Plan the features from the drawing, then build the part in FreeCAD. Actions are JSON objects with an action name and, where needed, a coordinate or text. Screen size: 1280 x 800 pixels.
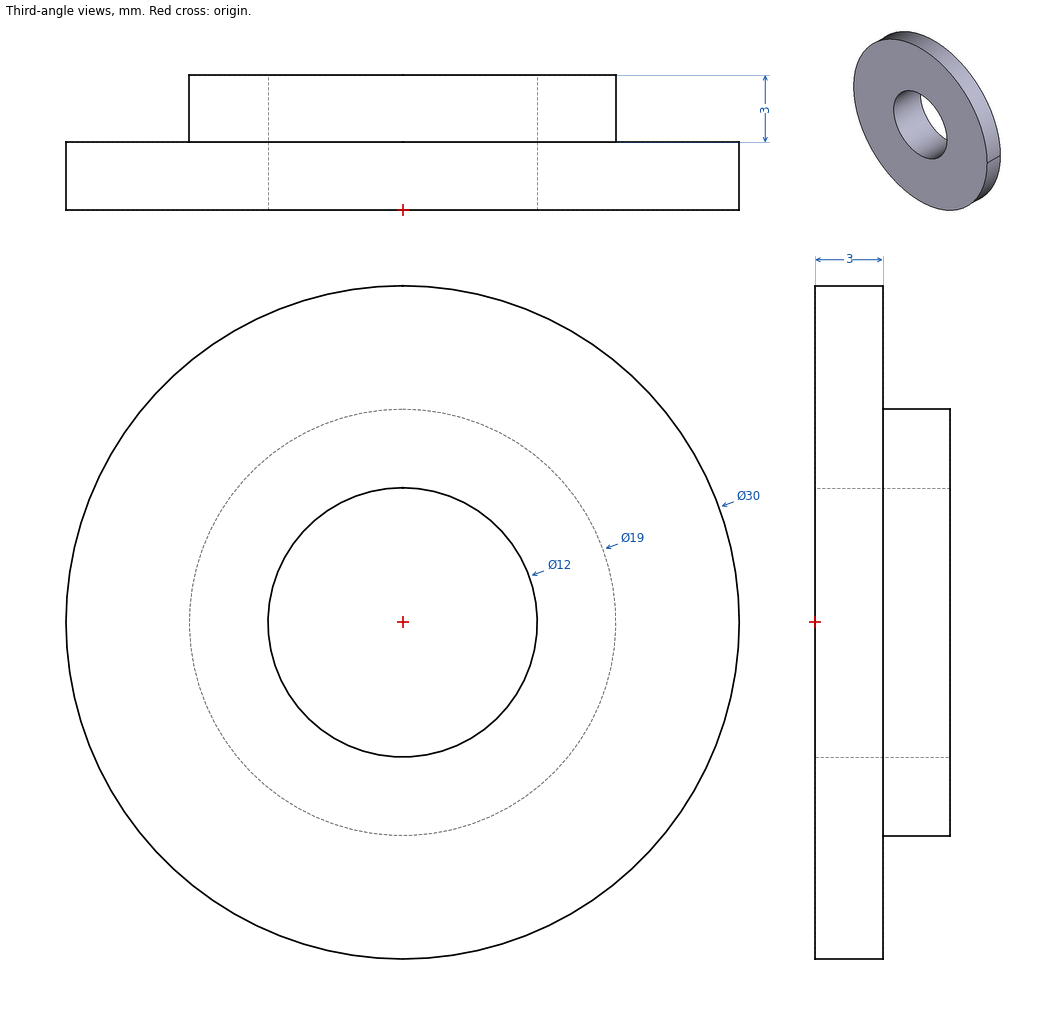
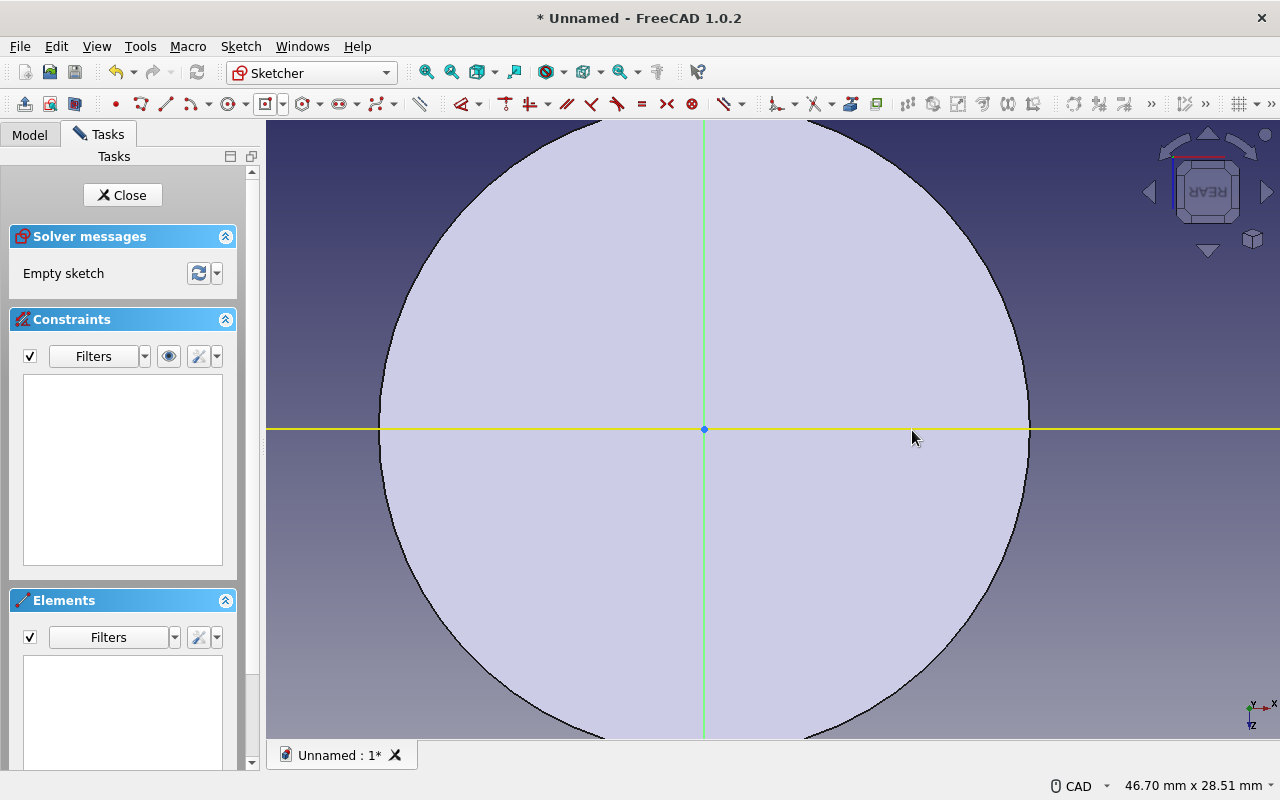
{"action": "left_click", "coordinate": [228, 104]}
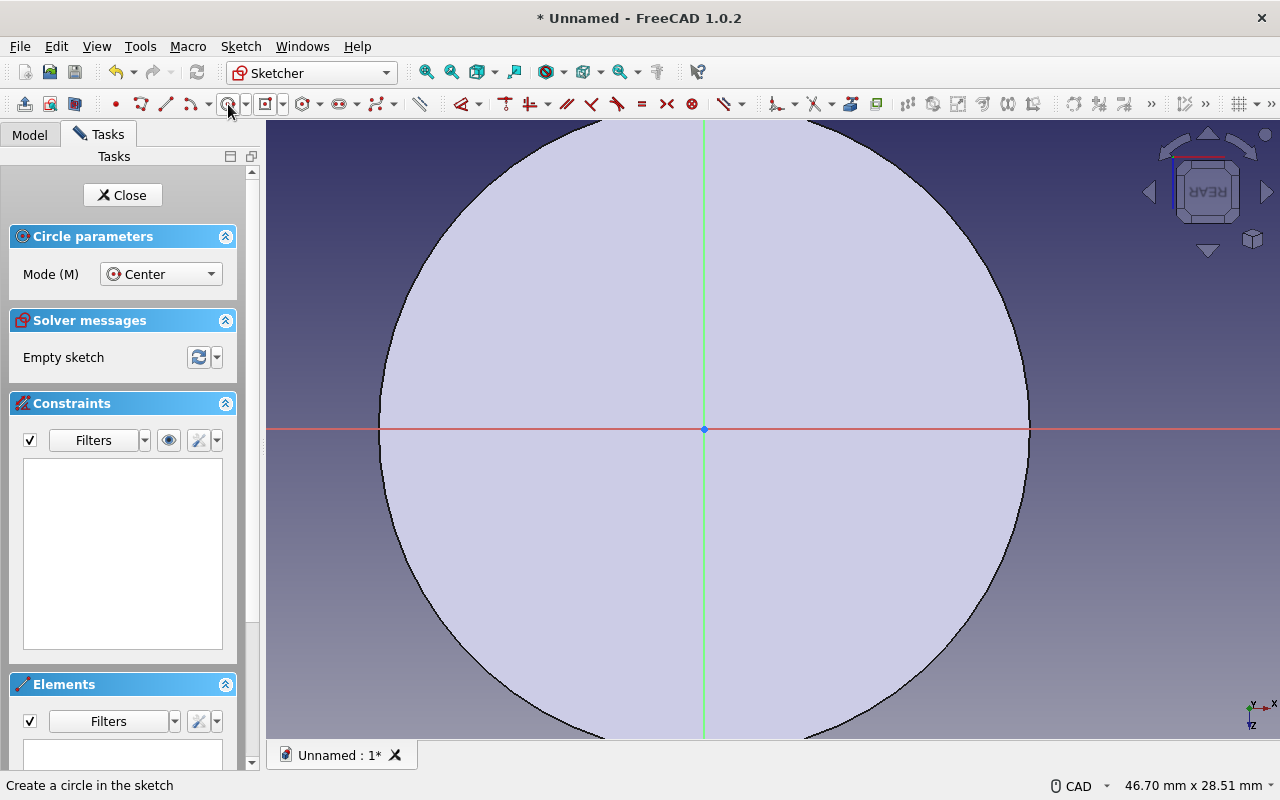
{"action": "left_click", "coordinate": [704, 429]}
{"action": "left_click", "coordinate": [850, 283]}
{"action": "key", "text": "Escape"}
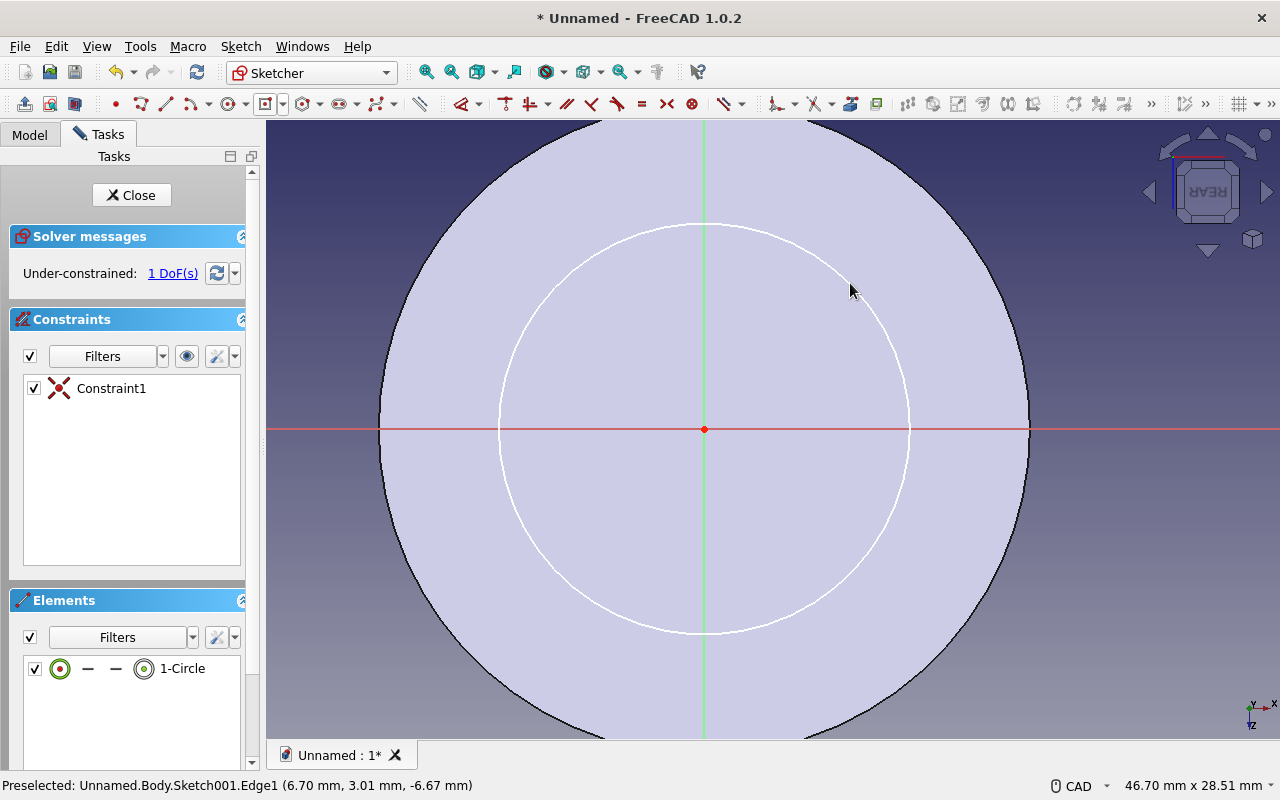
{"action": "left_click", "coordinate": [460, 104]}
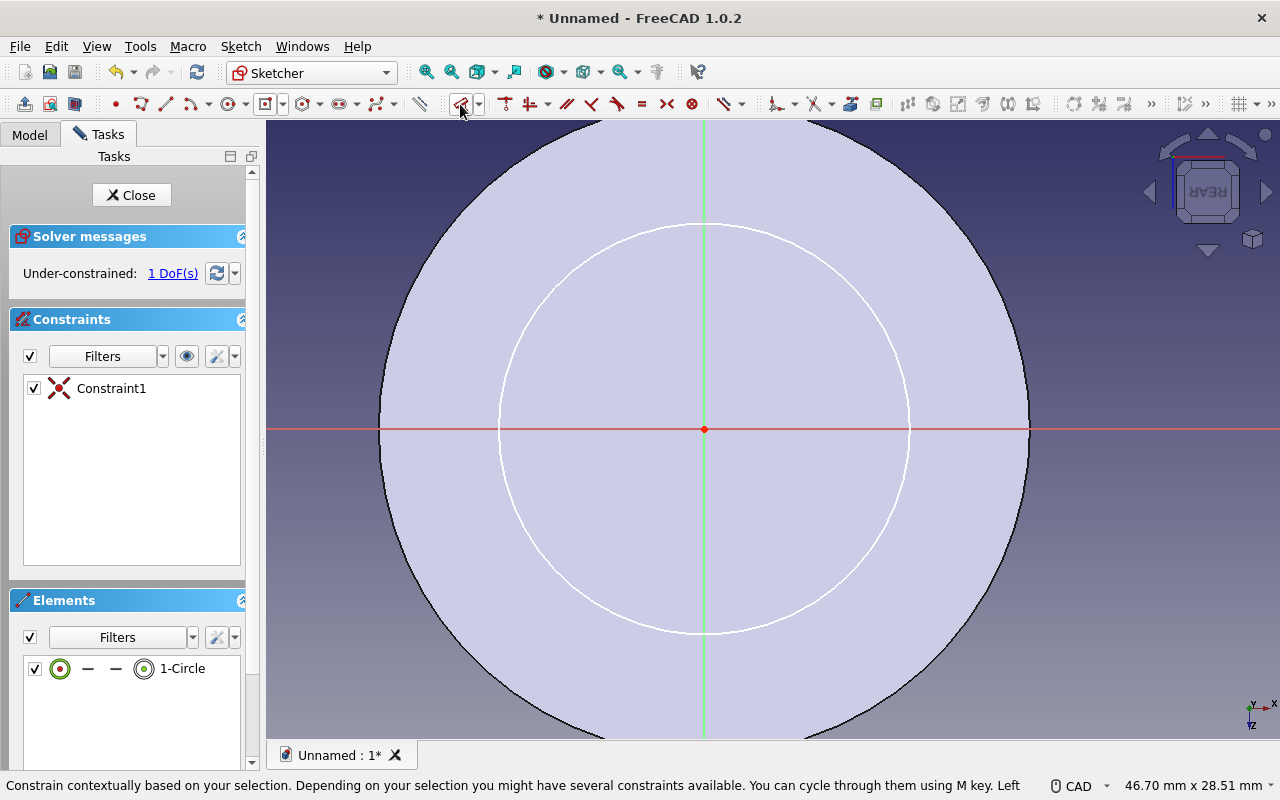
{"action": "left_click", "coordinate": [849, 283]}
{"action": "left_click", "coordinate": [872, 260]}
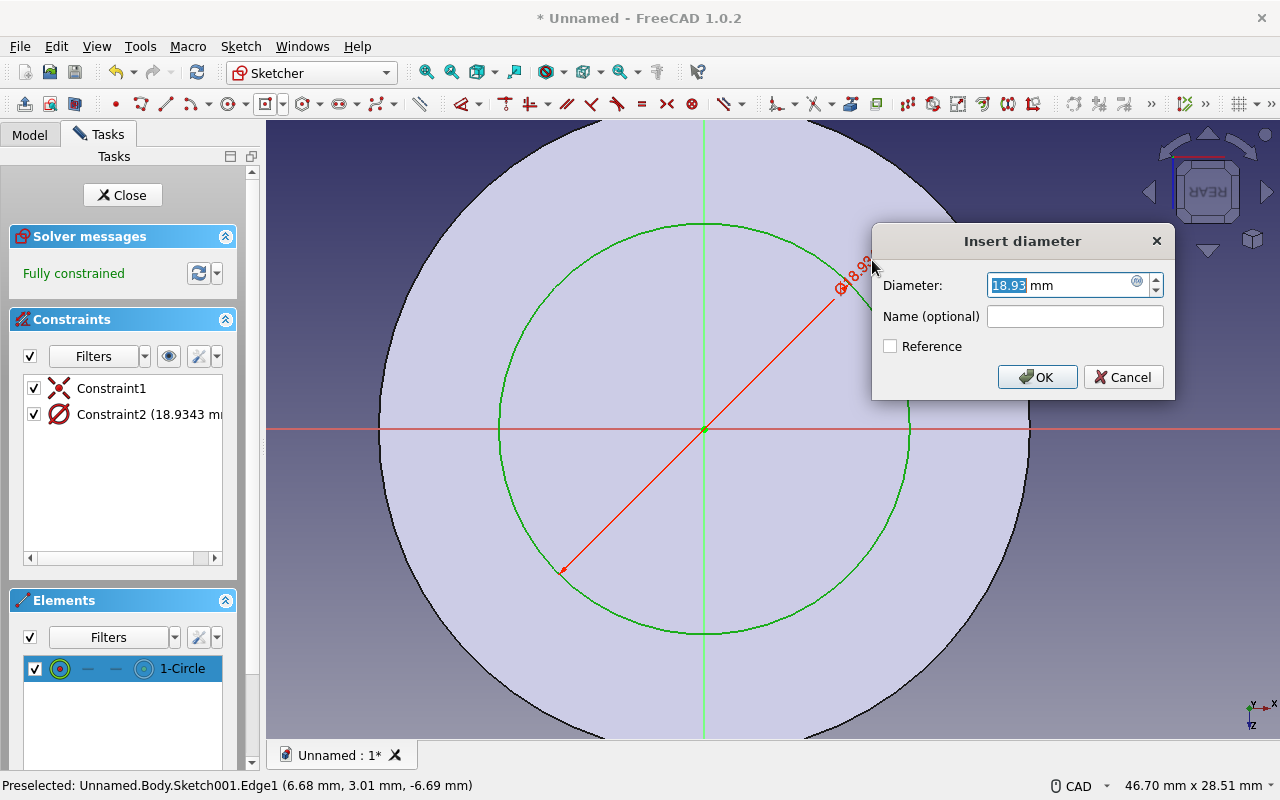
{"action": "type", "text": "19"}
{"action": "key", "text": "Return"}
{"action": "key", "text": "Escape"}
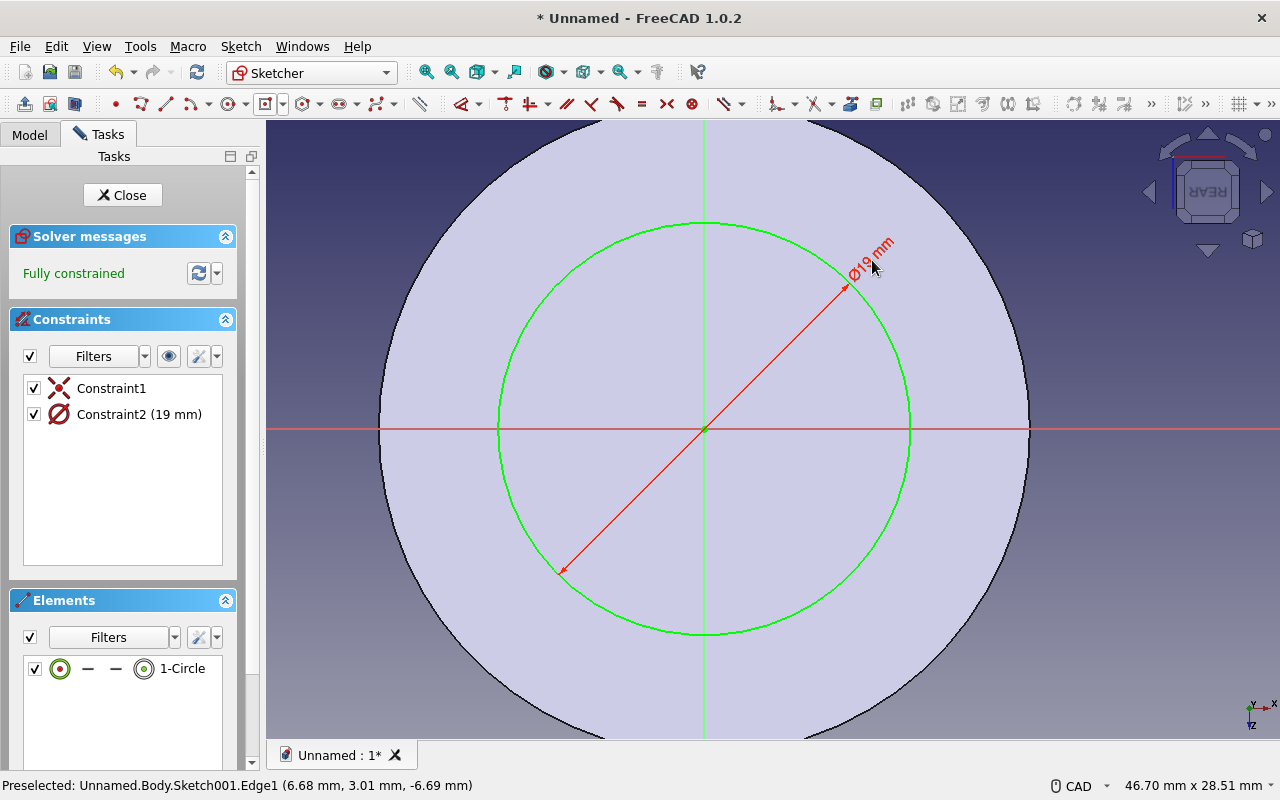
{"action": "left_click", "coordinate": [123, 195]}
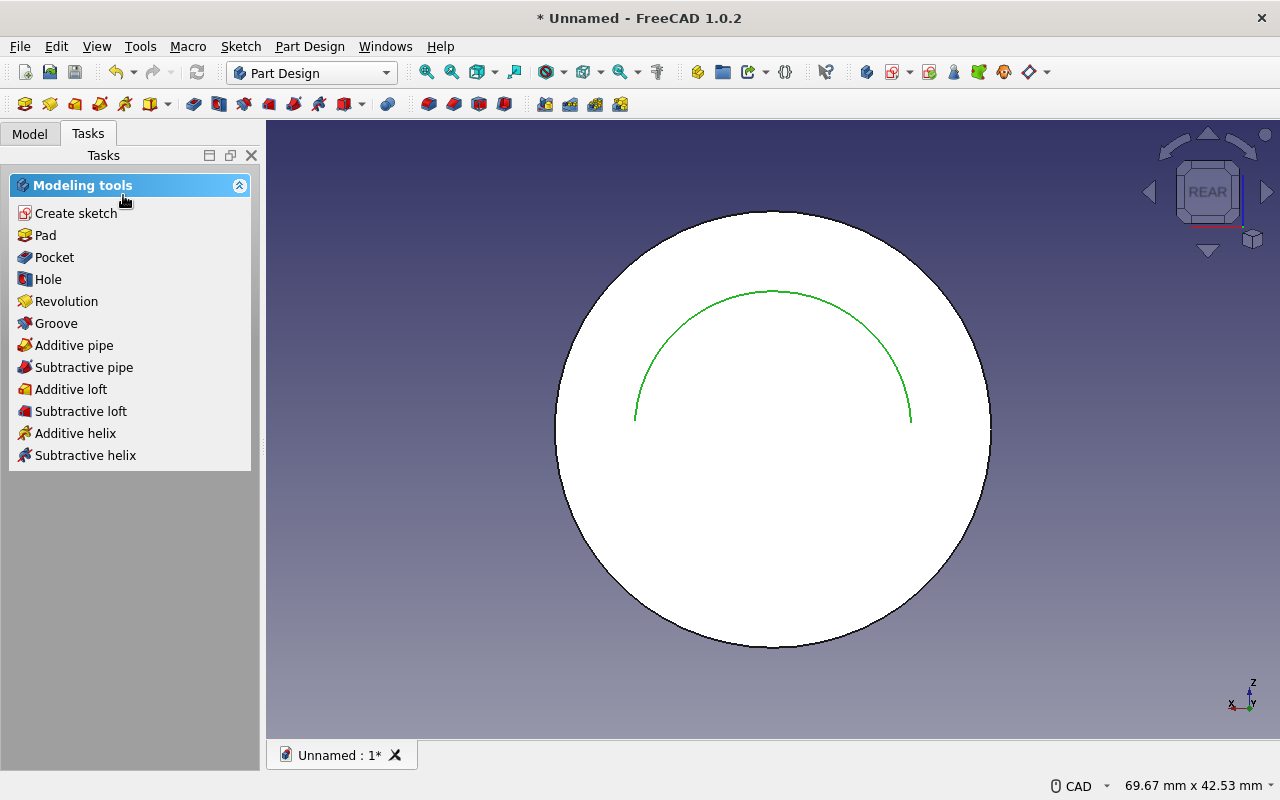
{"action": "left_click", "coordinate": [25, 104]}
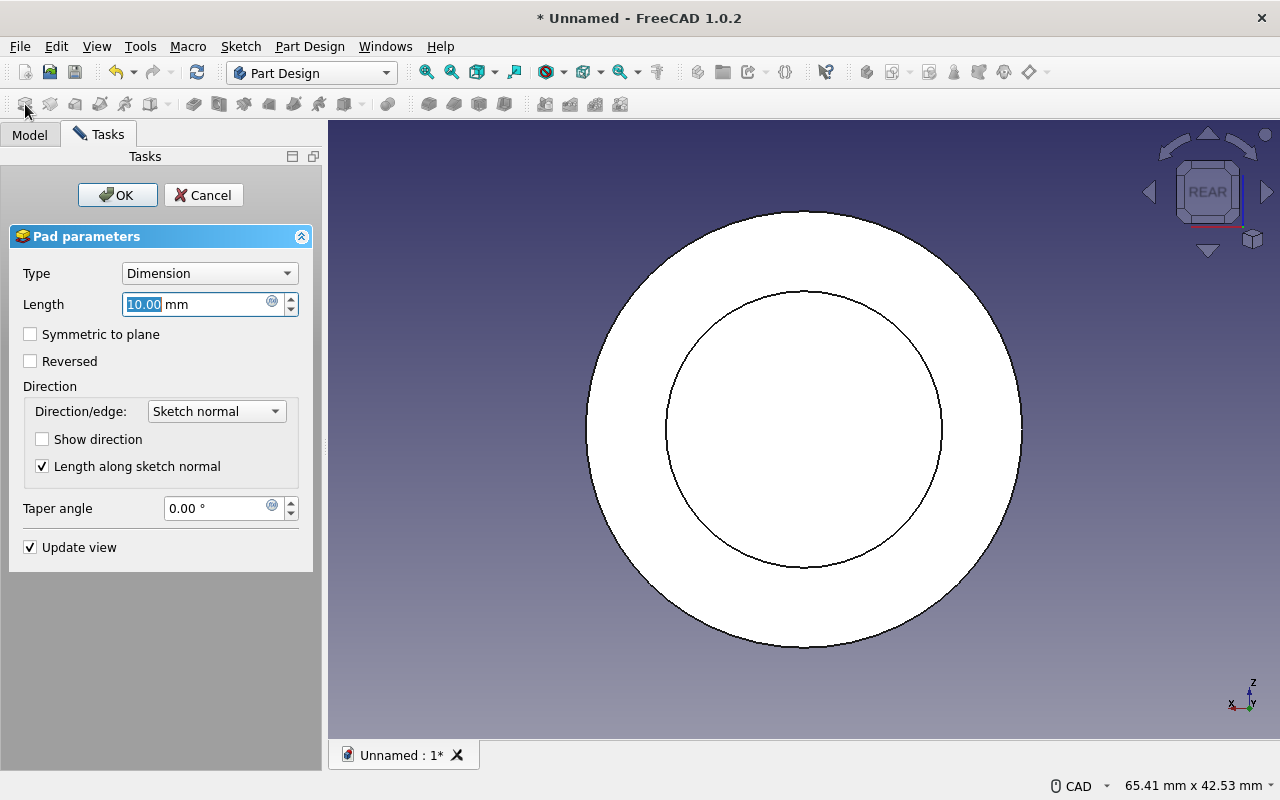
{"action": "type", "text": "3"}
{"action": "key", "text": "Tab"}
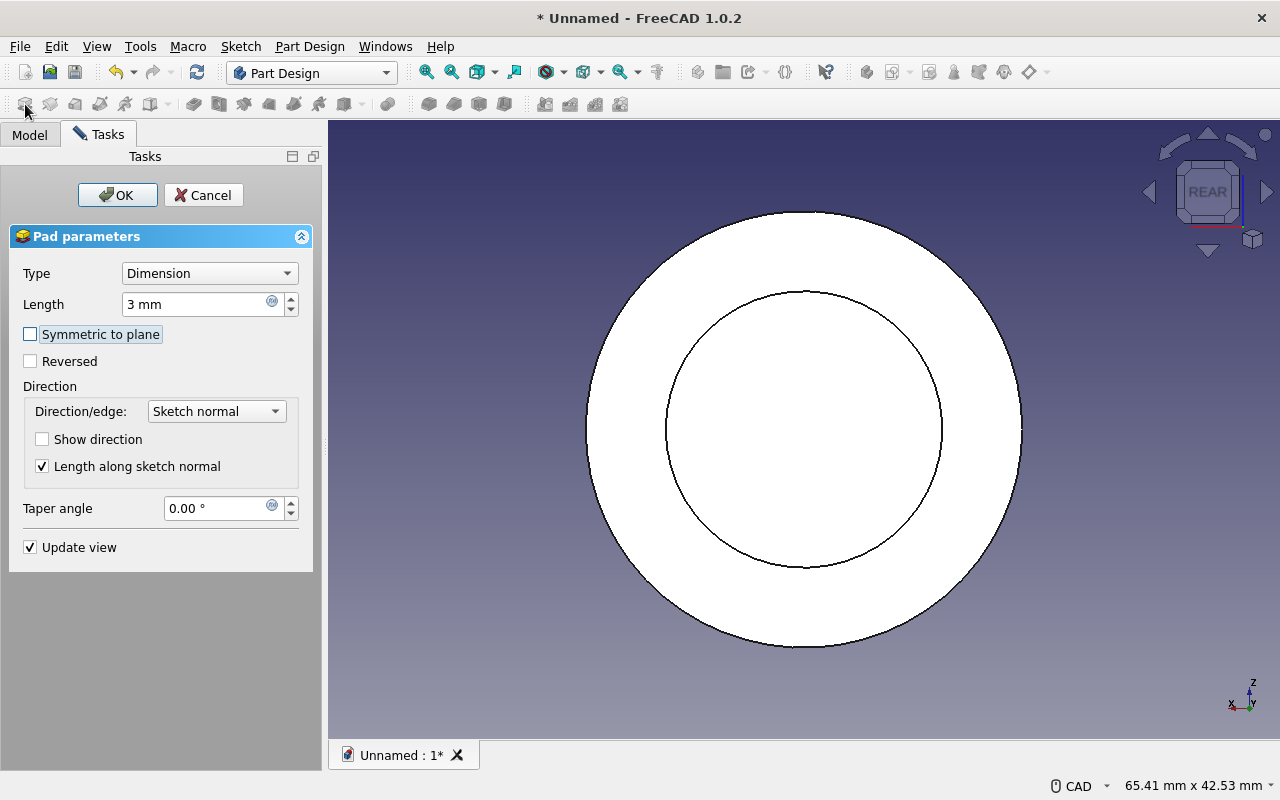
{"action": "left_click", "coordinate": [118, 195]}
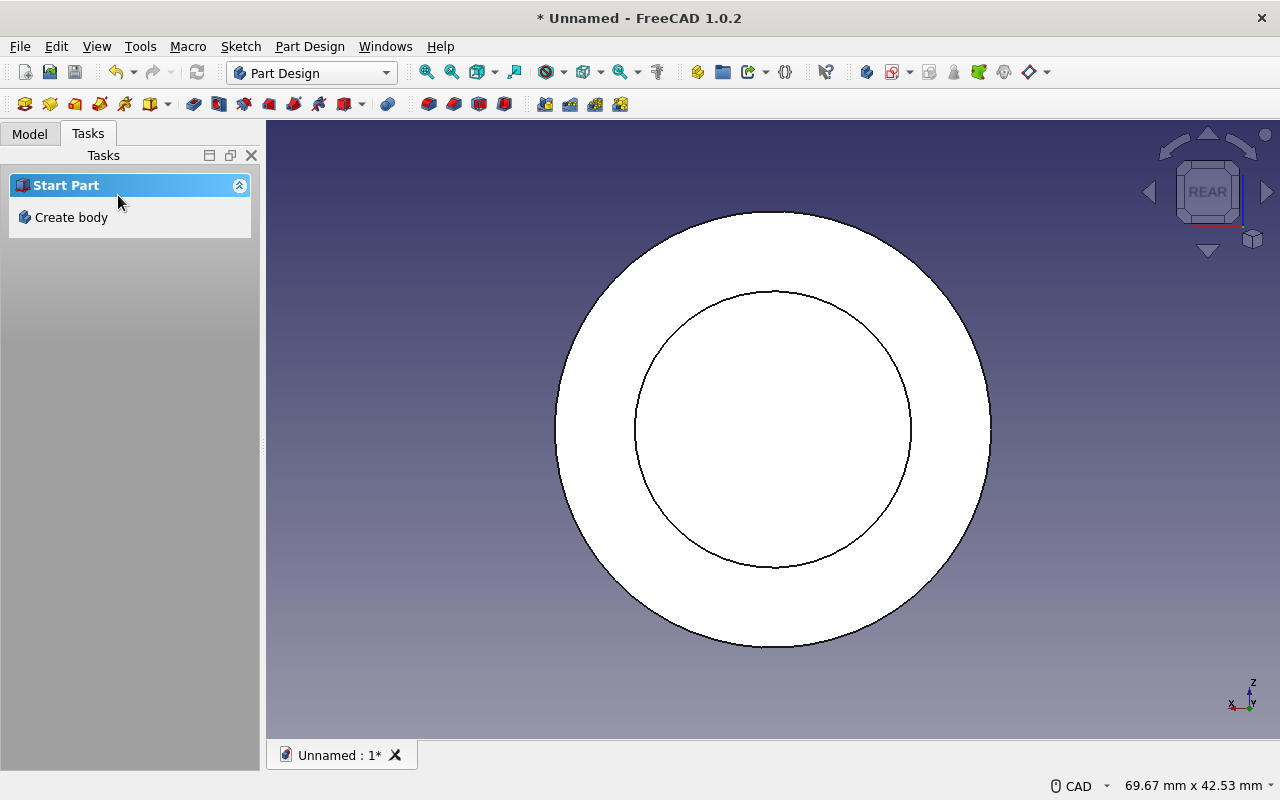
{"action": "left_click", "coordinate": [773, 428]}